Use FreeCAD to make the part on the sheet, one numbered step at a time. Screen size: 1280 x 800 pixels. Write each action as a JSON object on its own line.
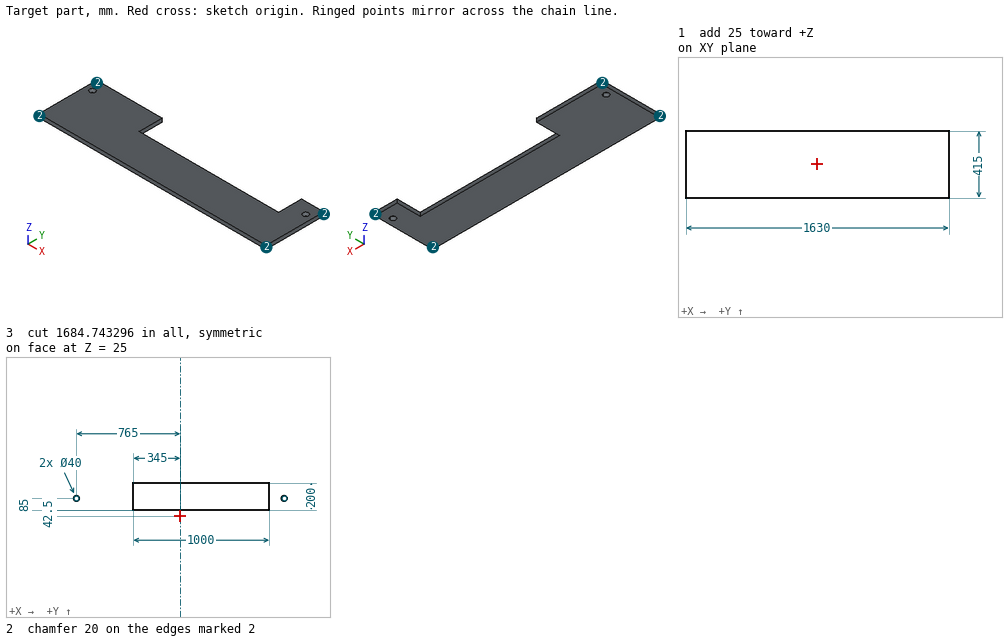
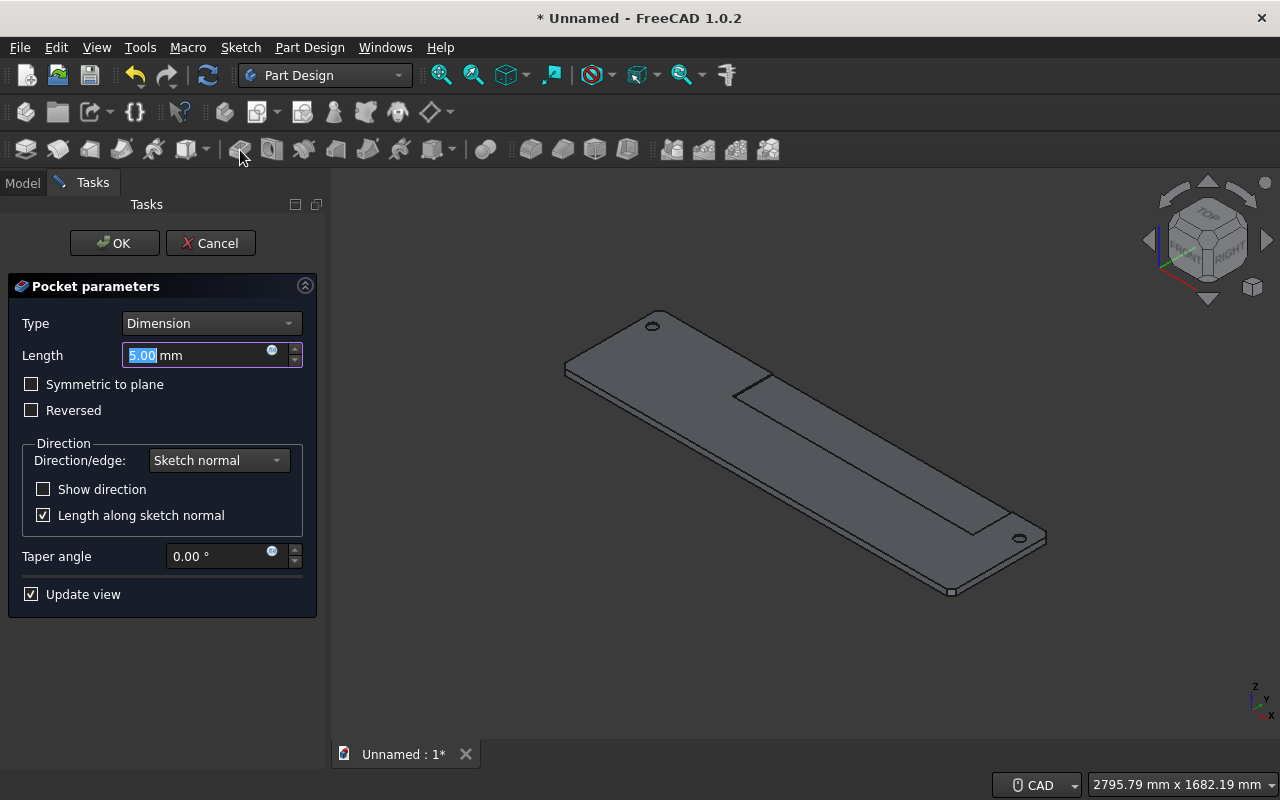
{"action": "type", "text": "1684.743296"}
{"action": "key", "text": "Tab"}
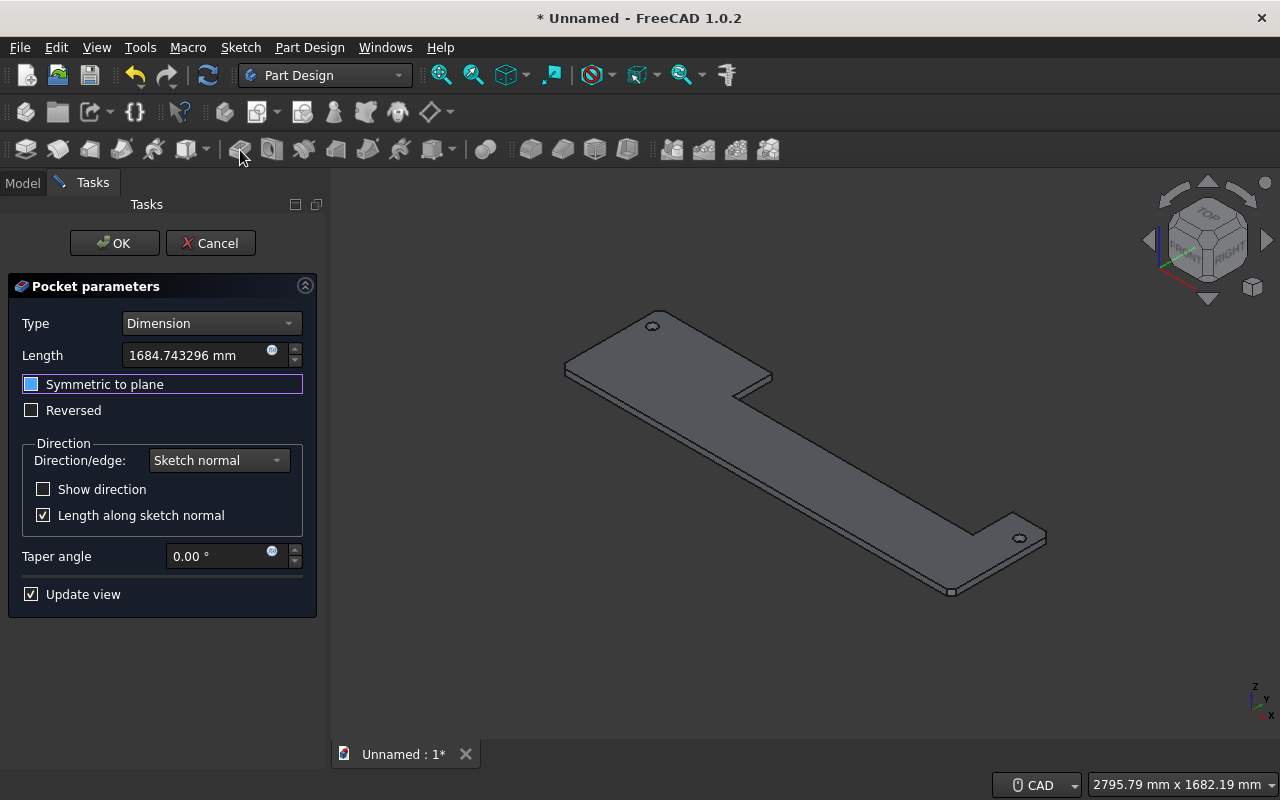
{"action": "left_click", "coordinate": [30, 384]}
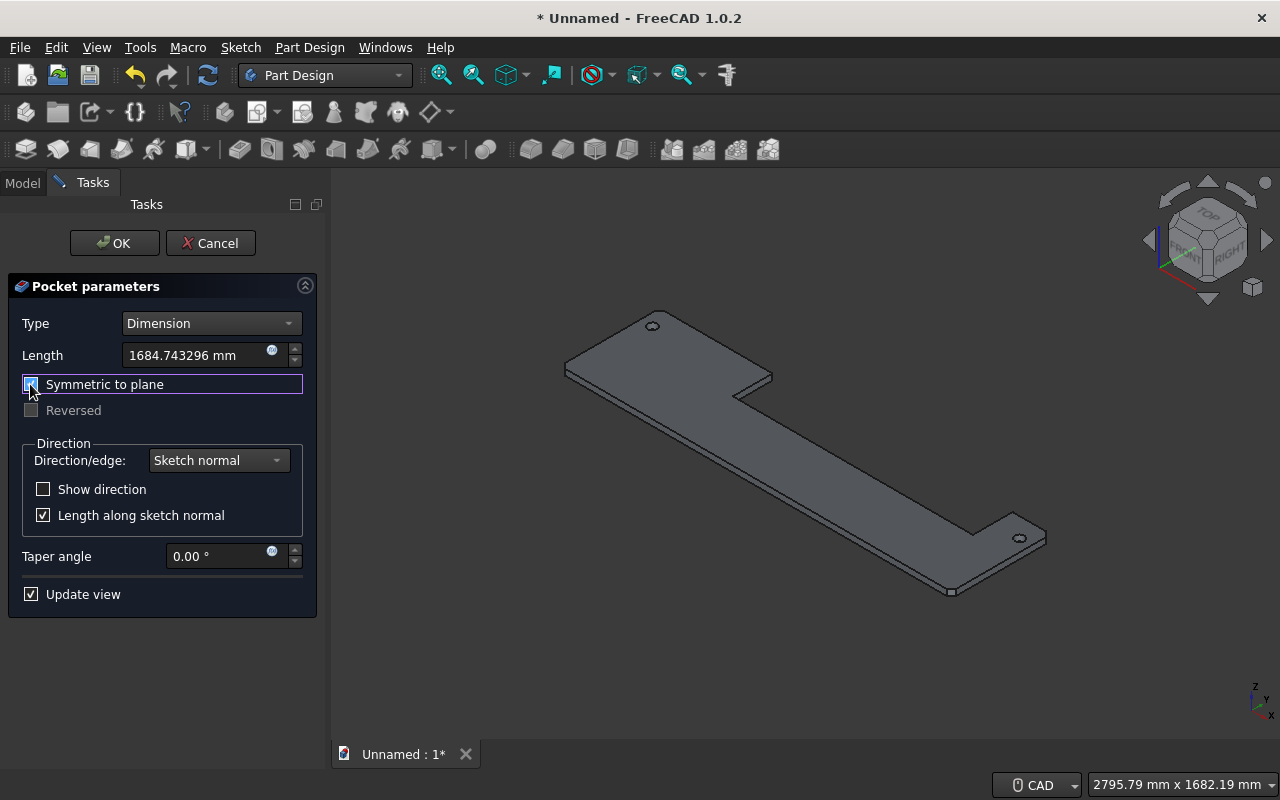
{"action": "left_click", "coordinate": [115, 243]}